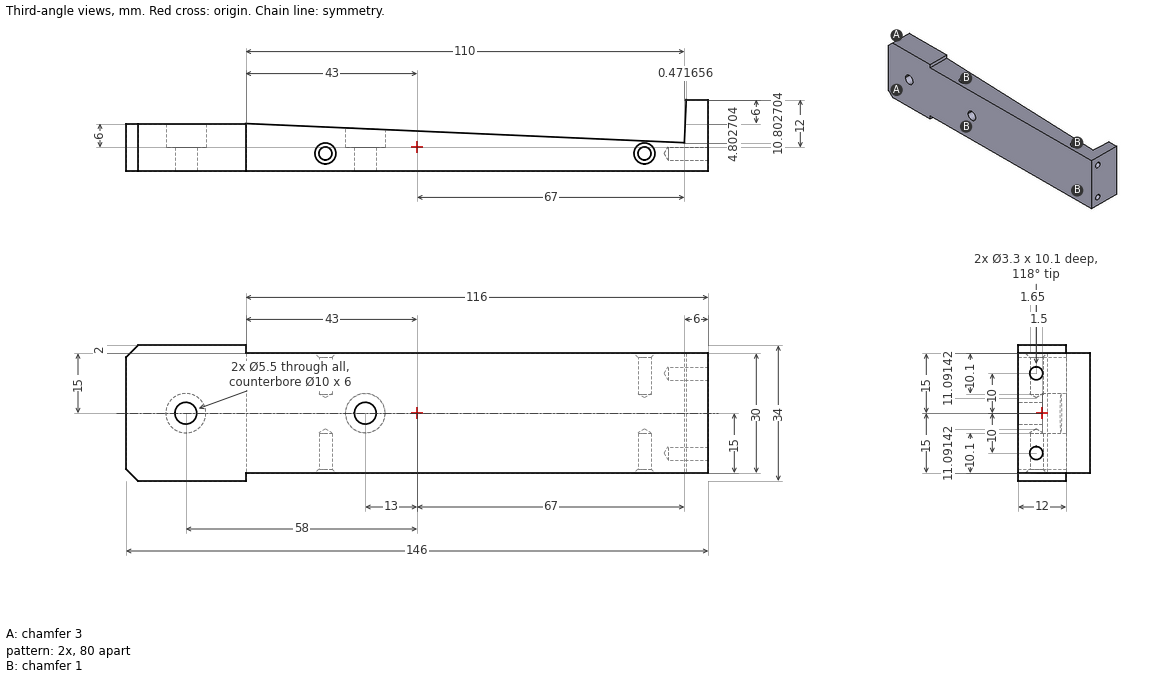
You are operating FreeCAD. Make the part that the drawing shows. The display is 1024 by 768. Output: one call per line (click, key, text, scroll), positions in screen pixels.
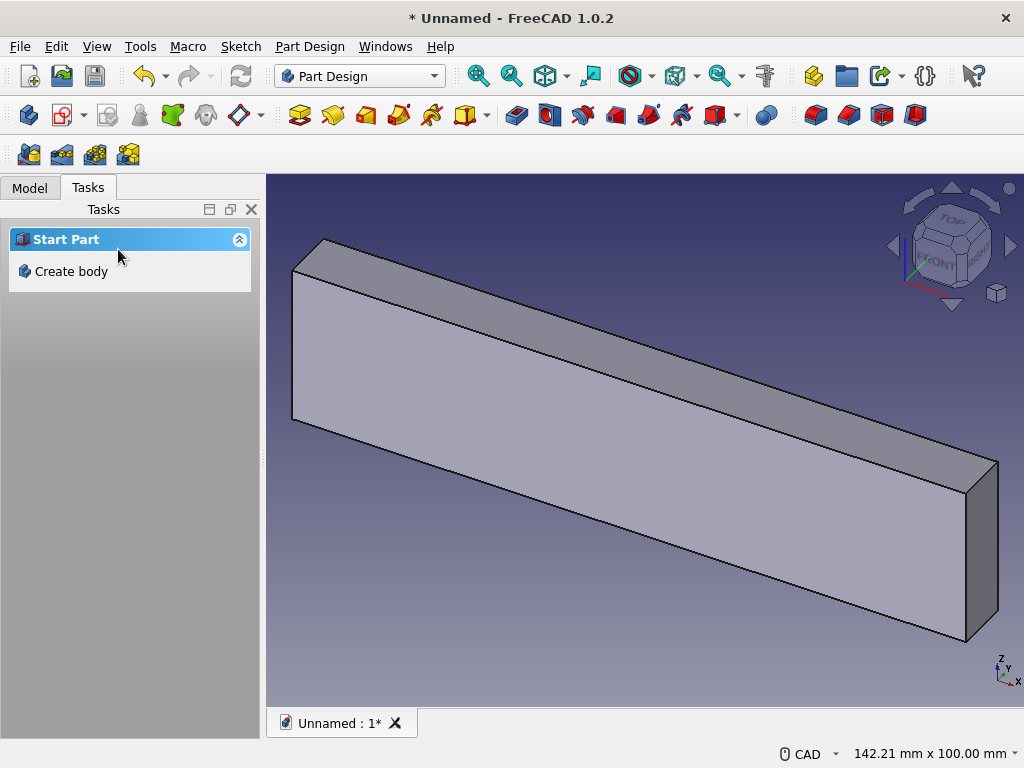
key(4)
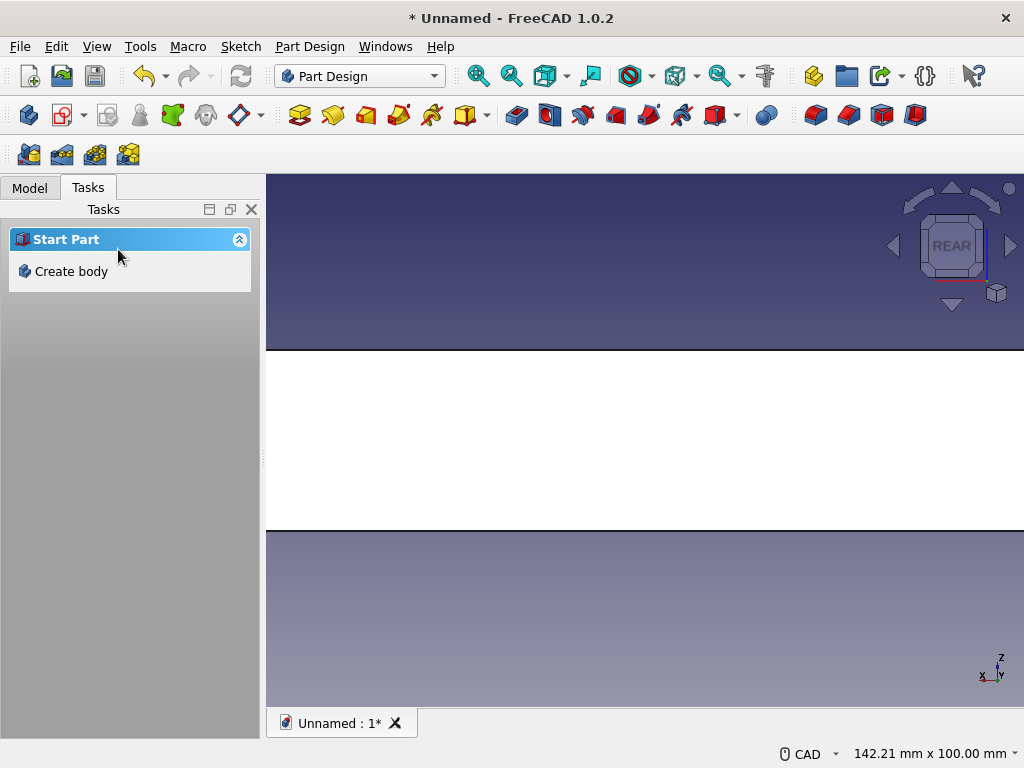
click(479, 76)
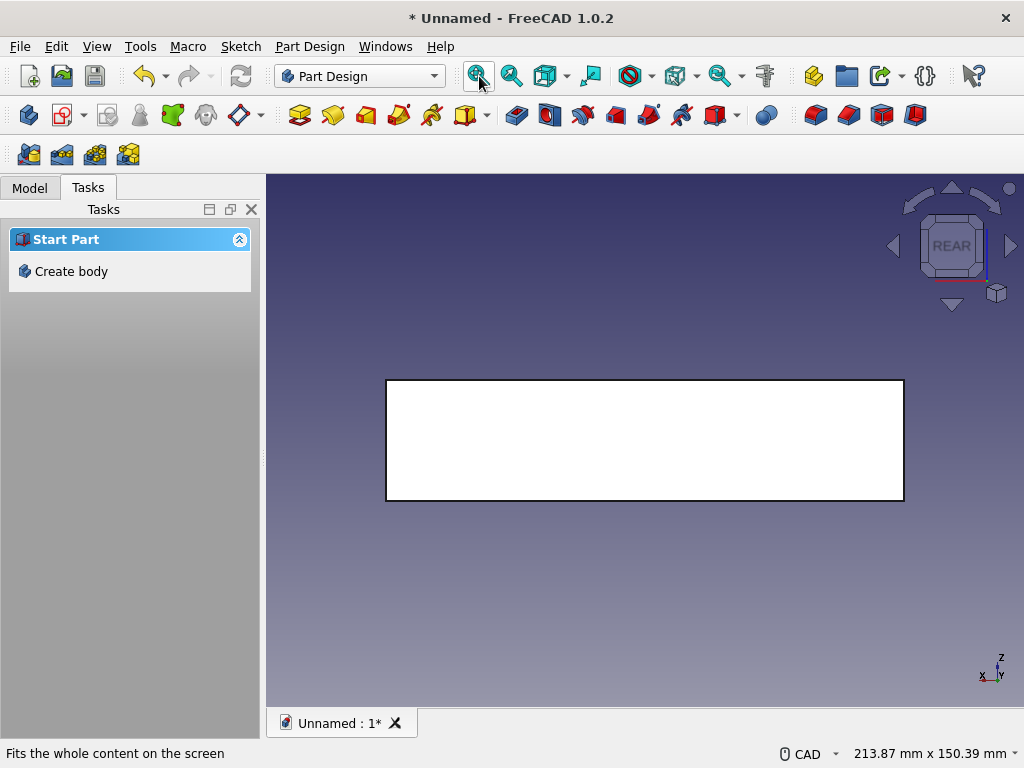
click(497, 440)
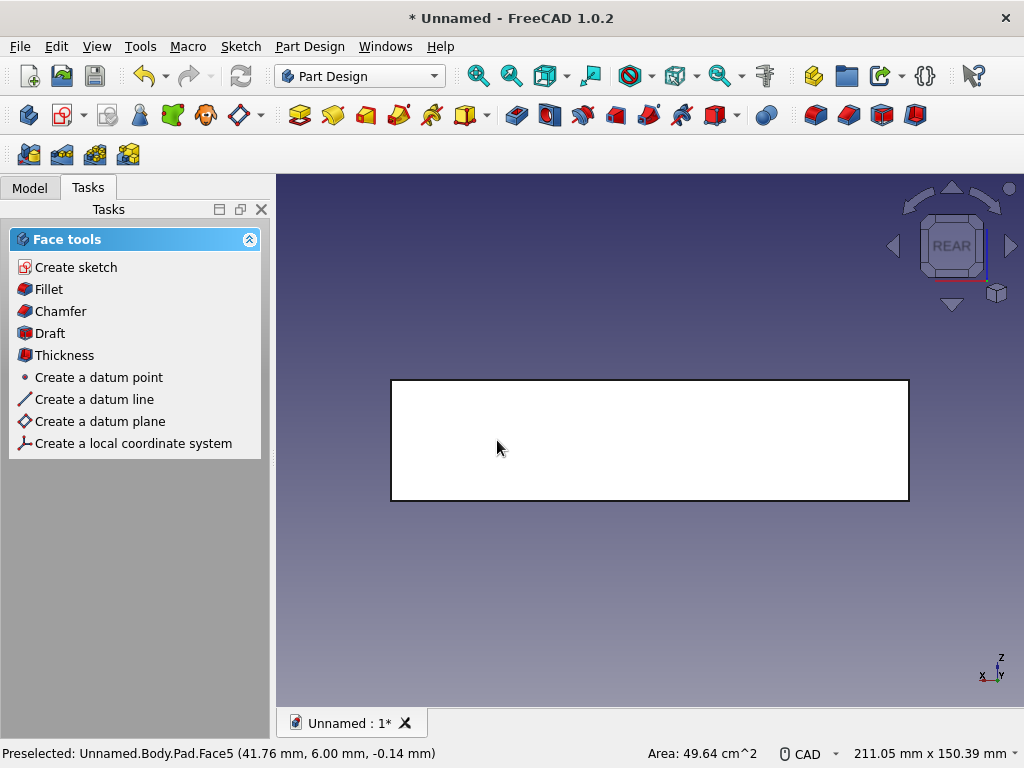
click(62, 116)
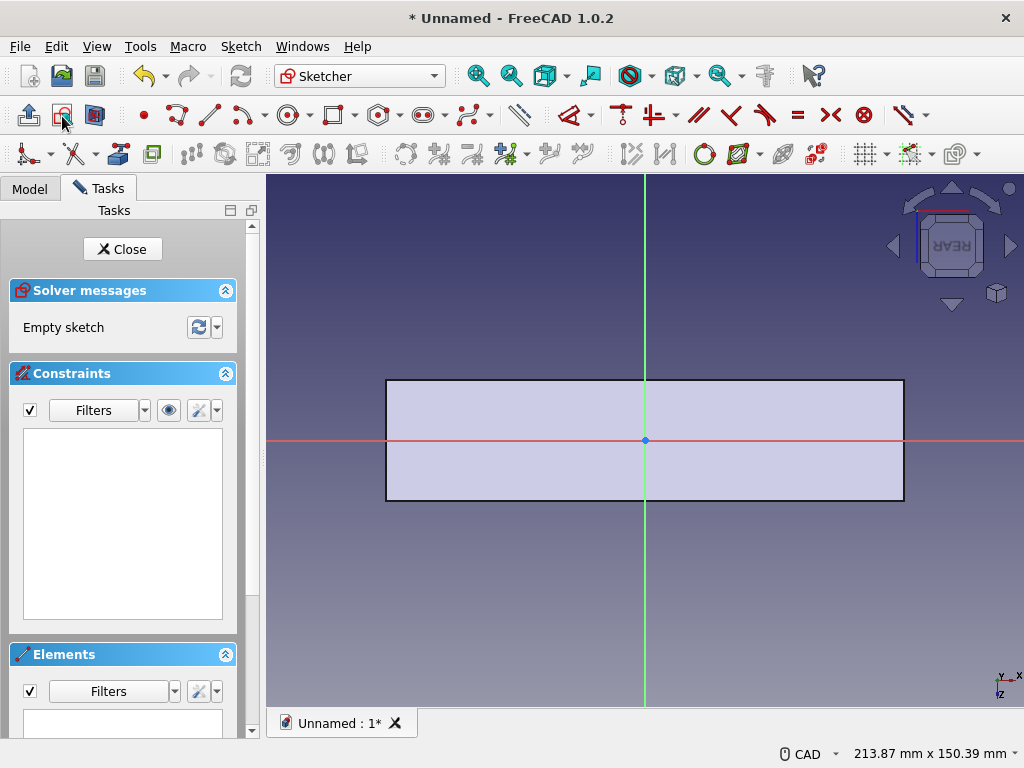
scroll(490, 441, up, 3)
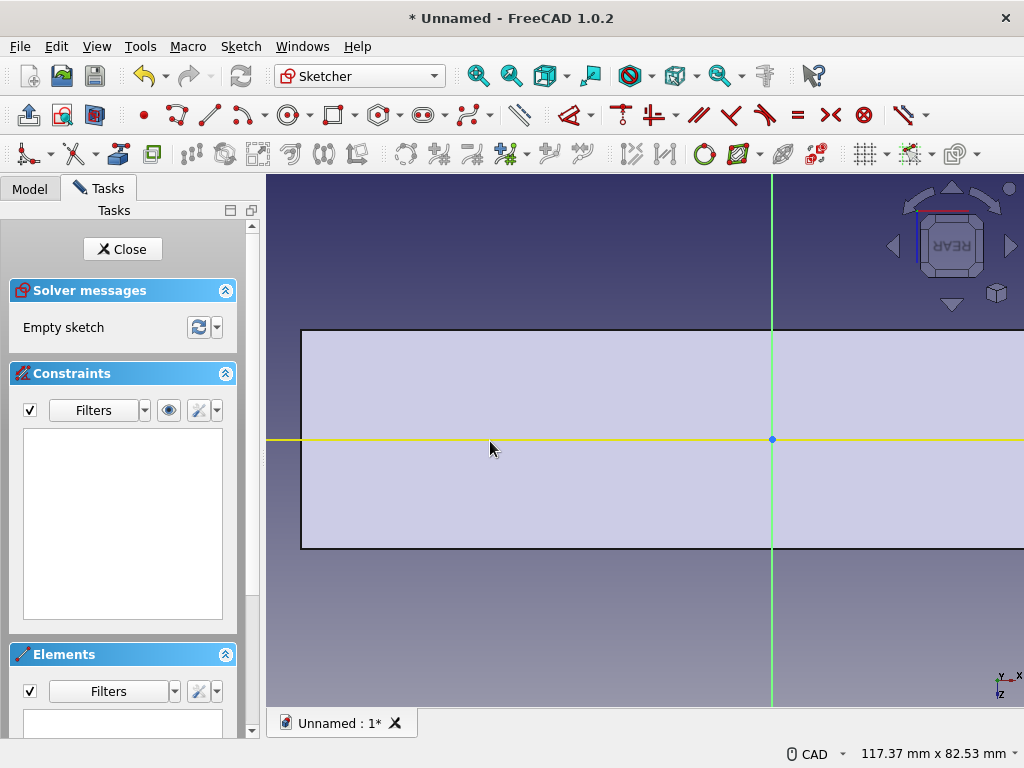
click(288, 116)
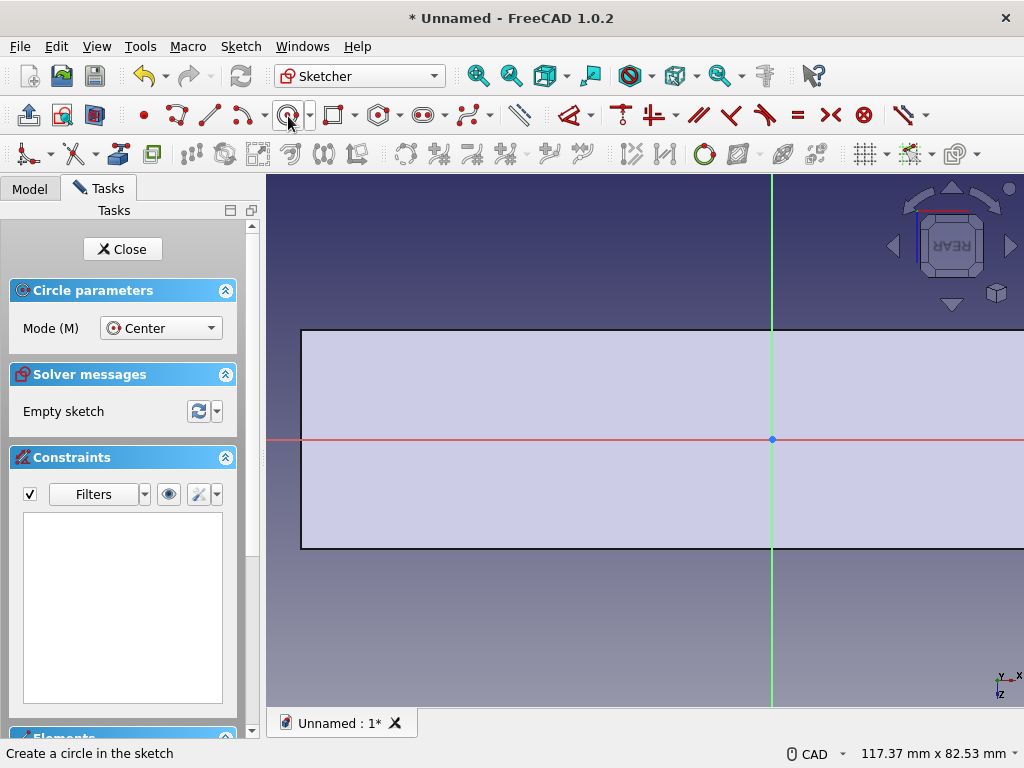
scroll(398, 440, up, 2)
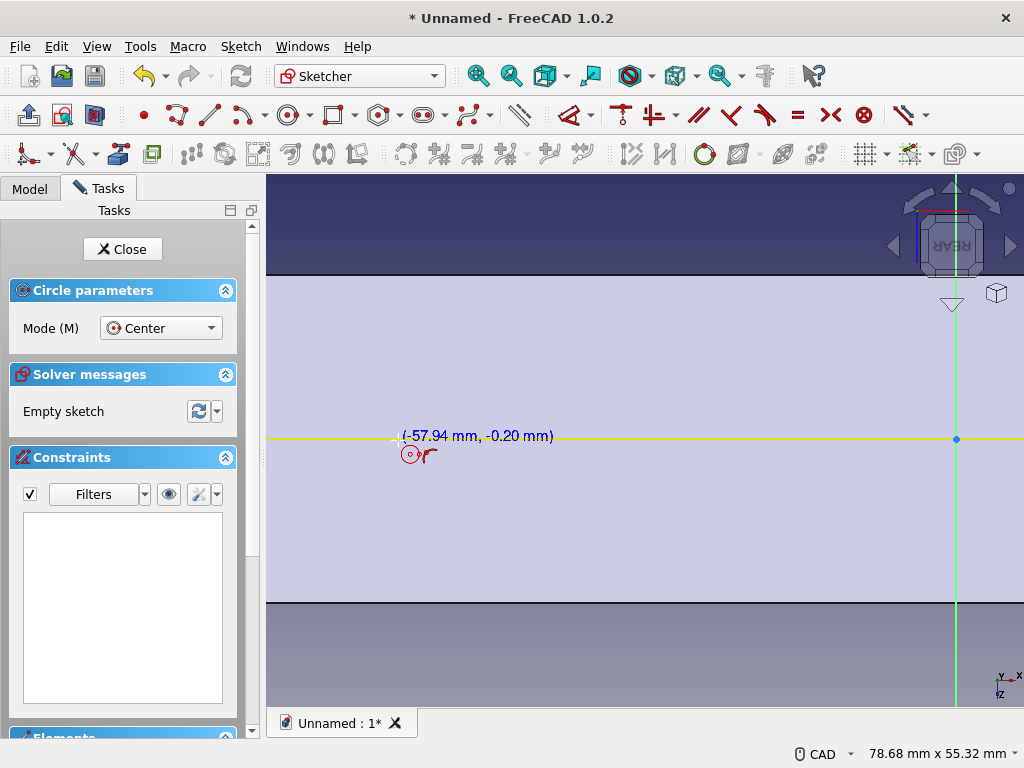
click(397, 439)
move(416, 421)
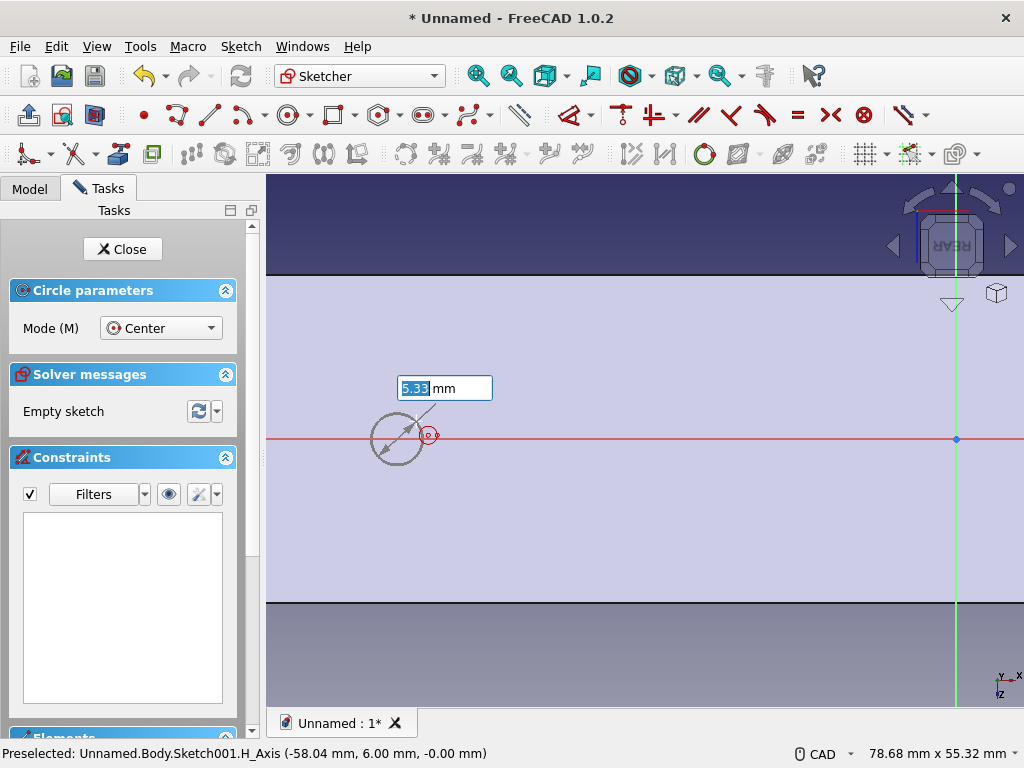
text(5.5)
key(Return)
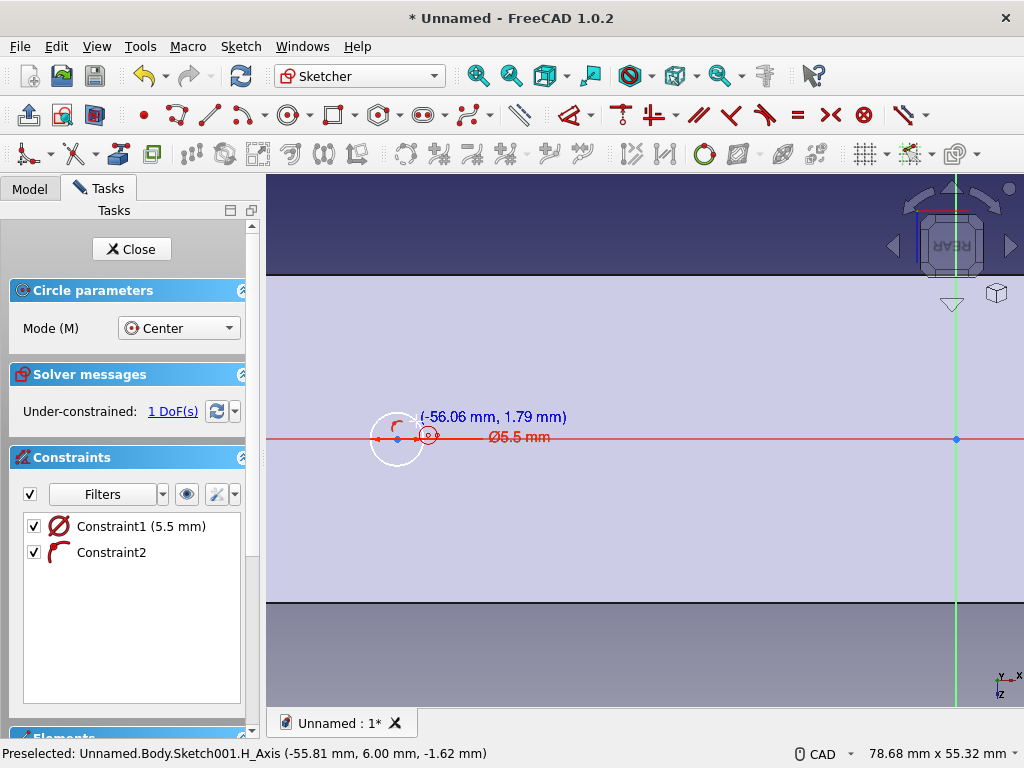
click(831, 439)
move(850, 421)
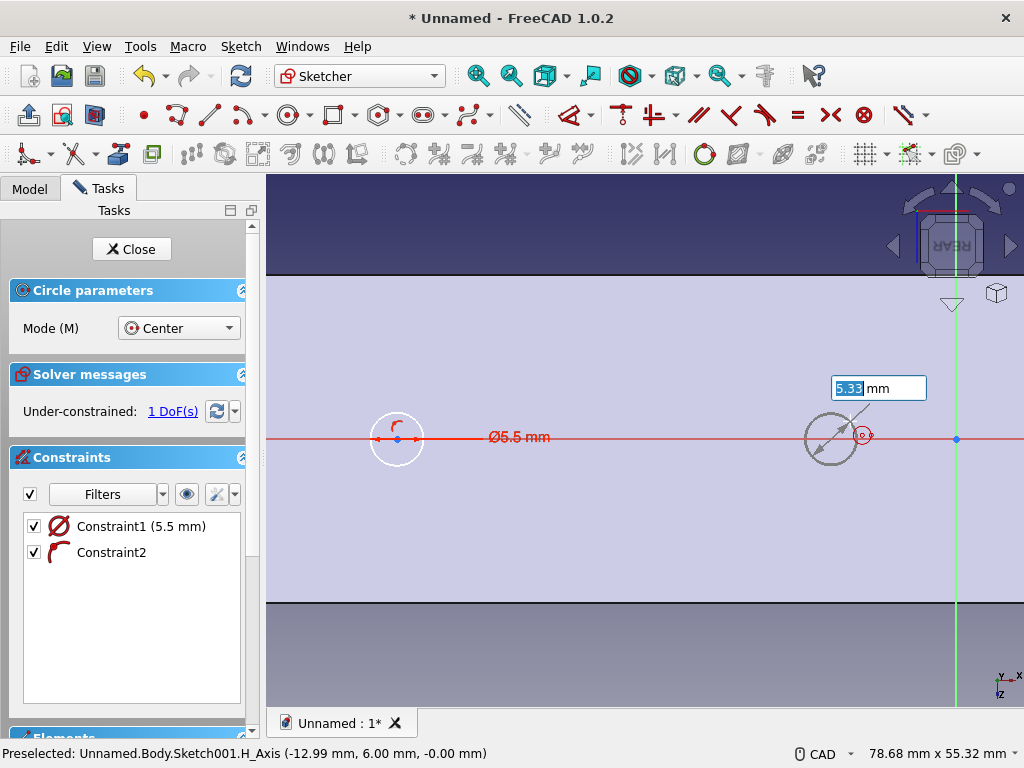
text(5.5)
key(Return)
key(Escape)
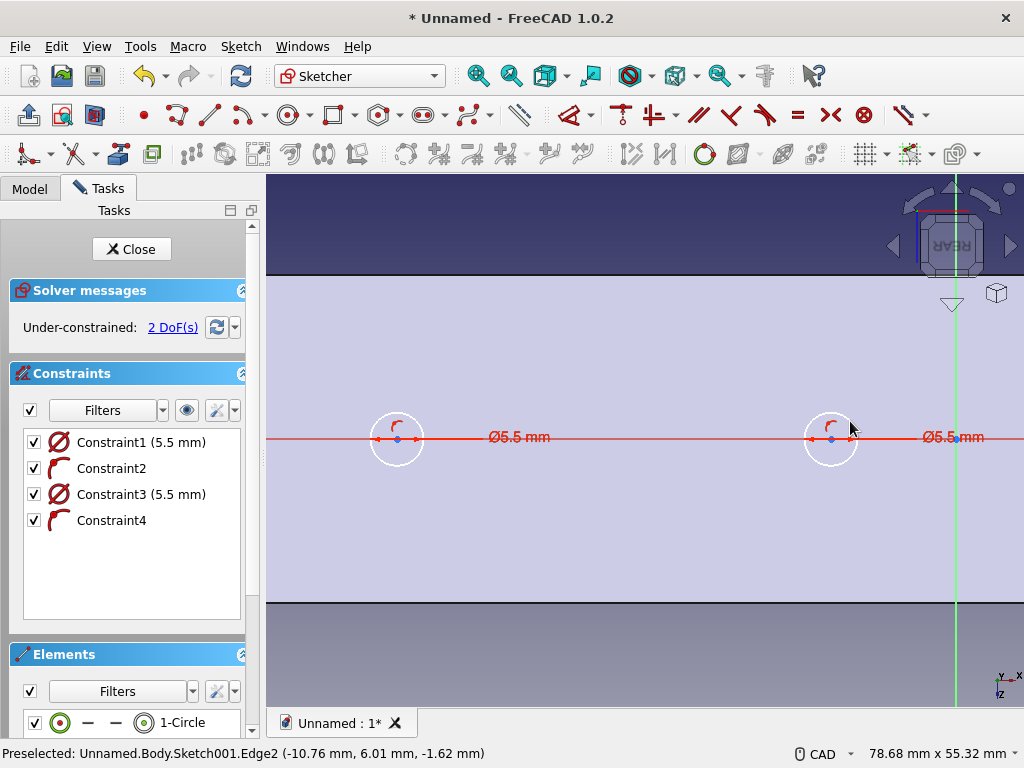
key(d)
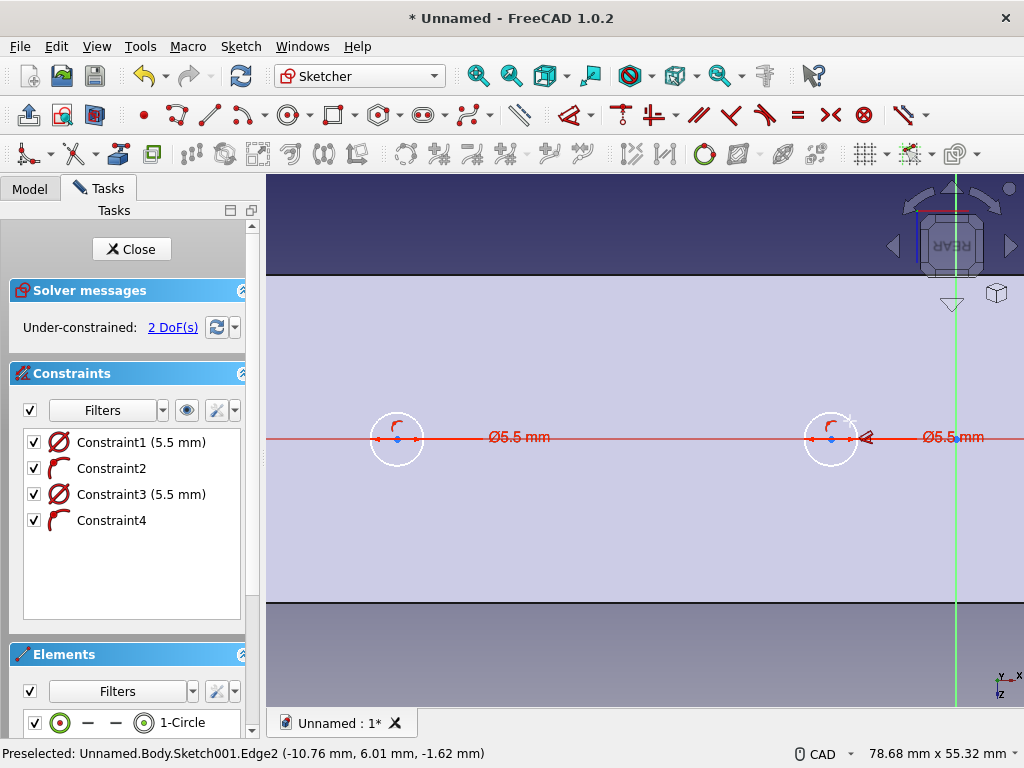
click(397, 439)
click(628, 473)